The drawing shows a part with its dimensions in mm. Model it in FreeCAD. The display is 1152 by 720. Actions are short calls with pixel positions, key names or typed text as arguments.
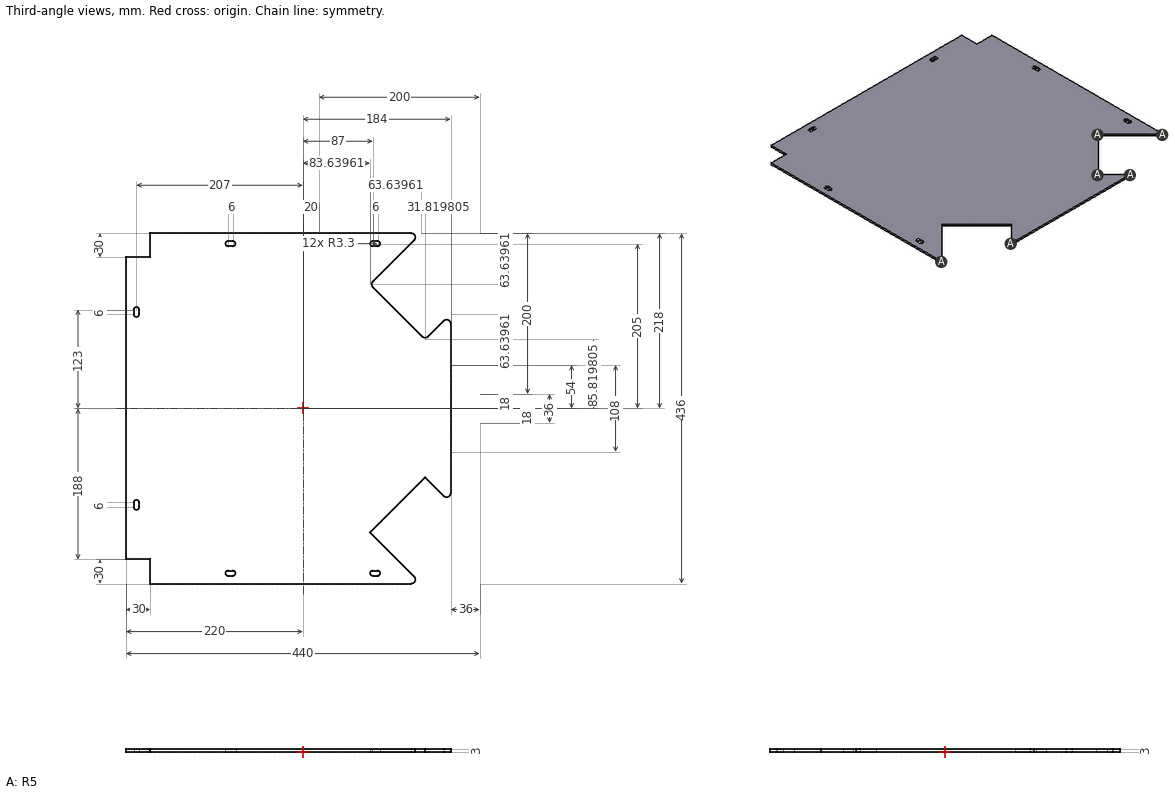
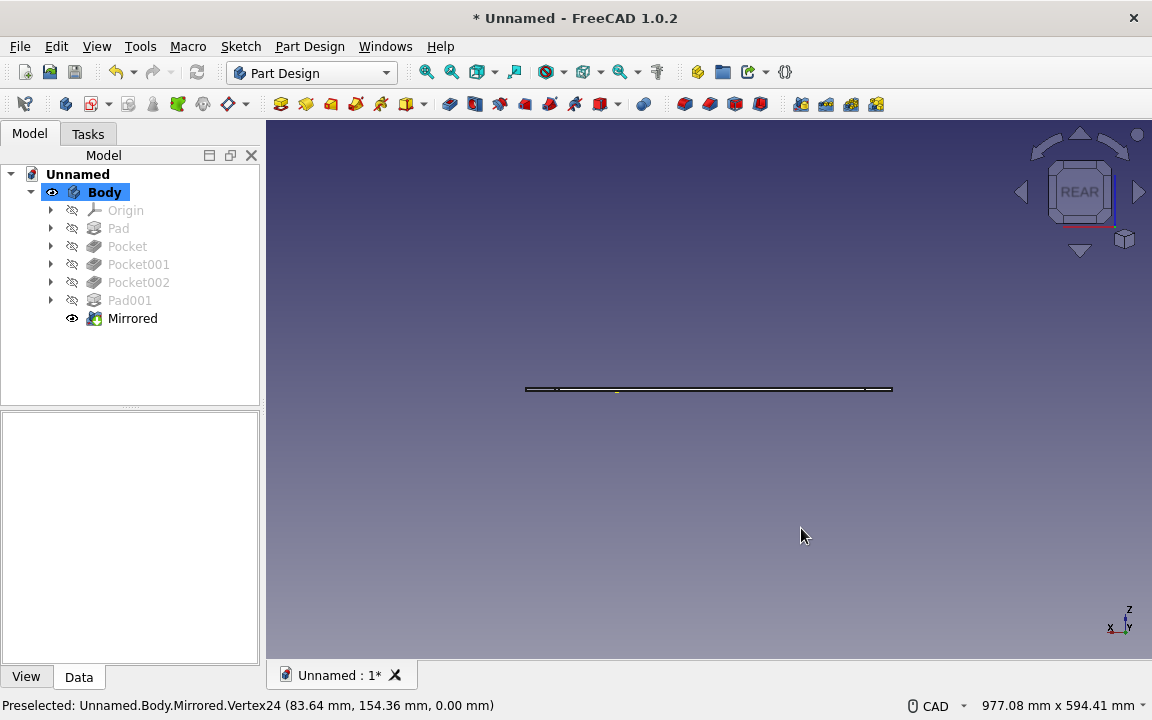
scroll(617, 389, up, 14)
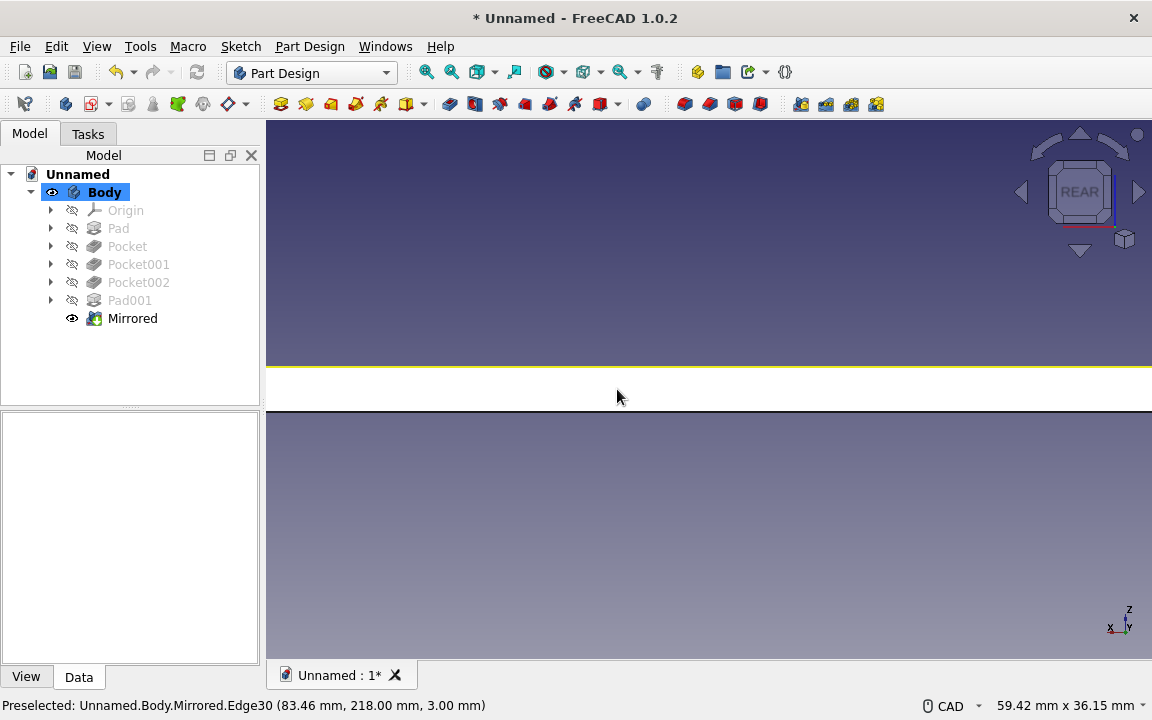
key(v)
key(f)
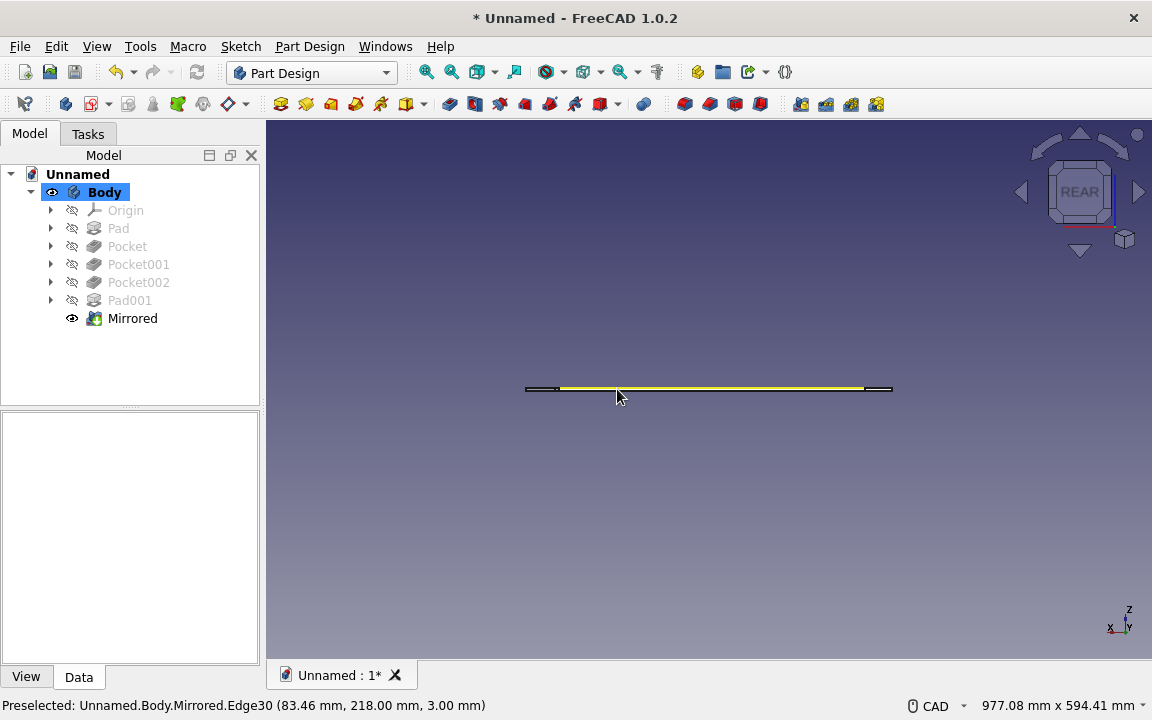
key(6)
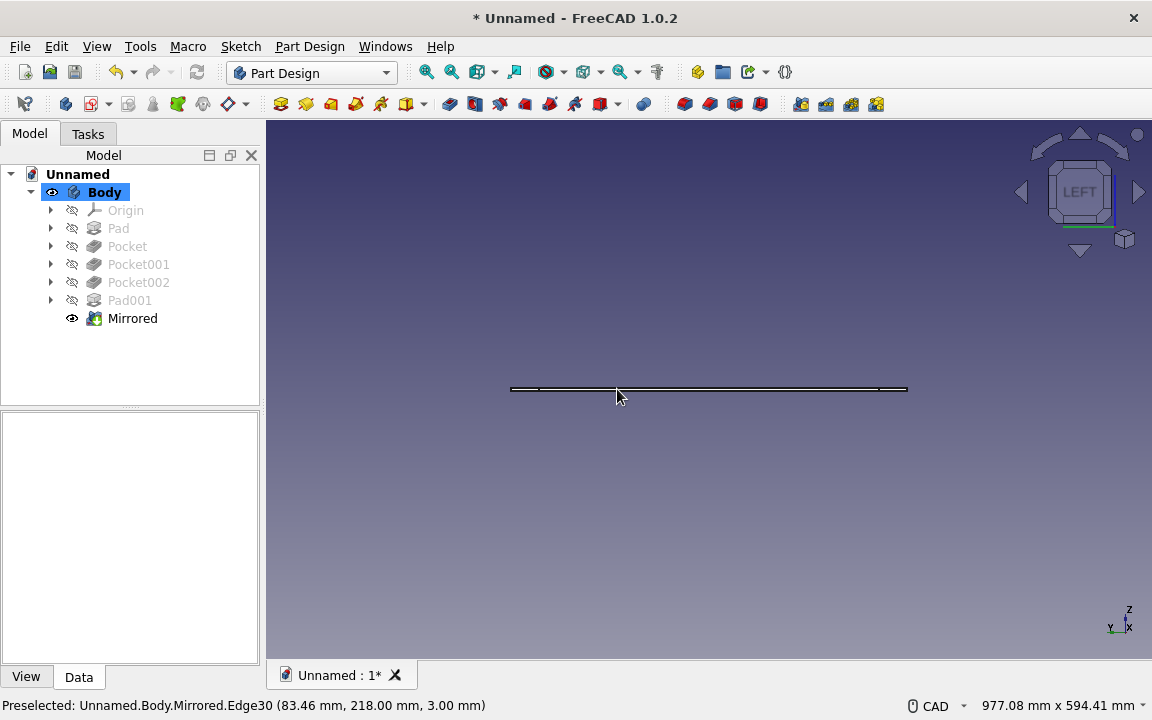
key(v)
key(f)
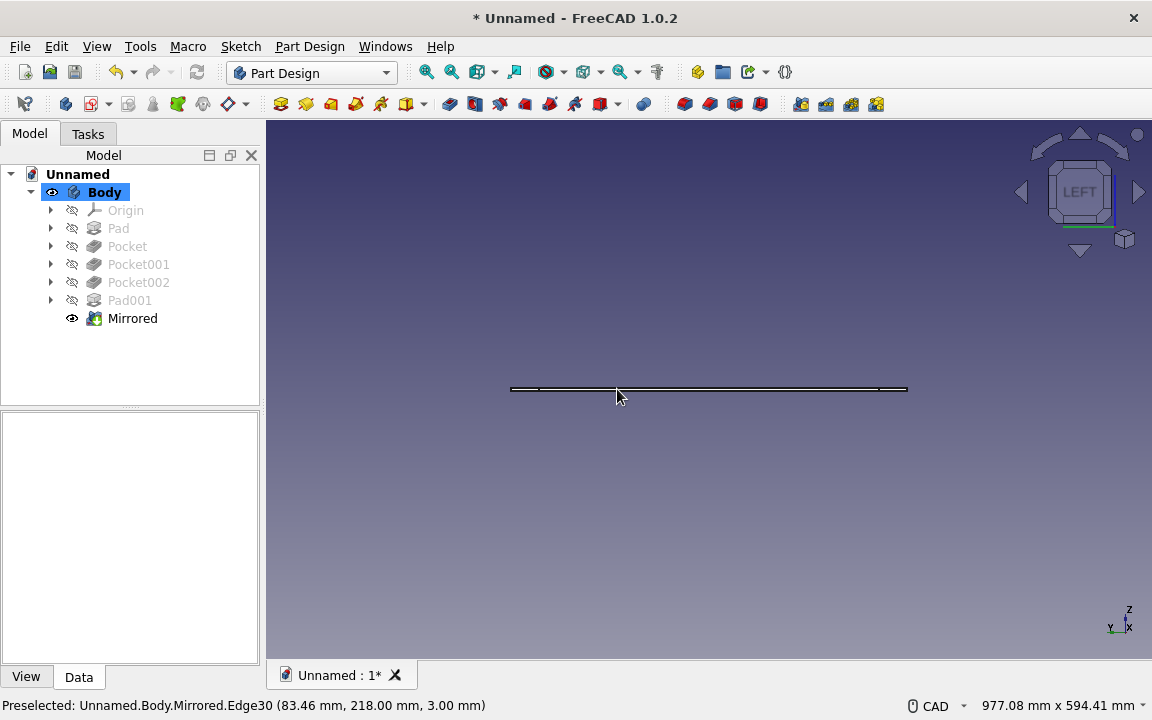
scroll(569, 388, up, 14)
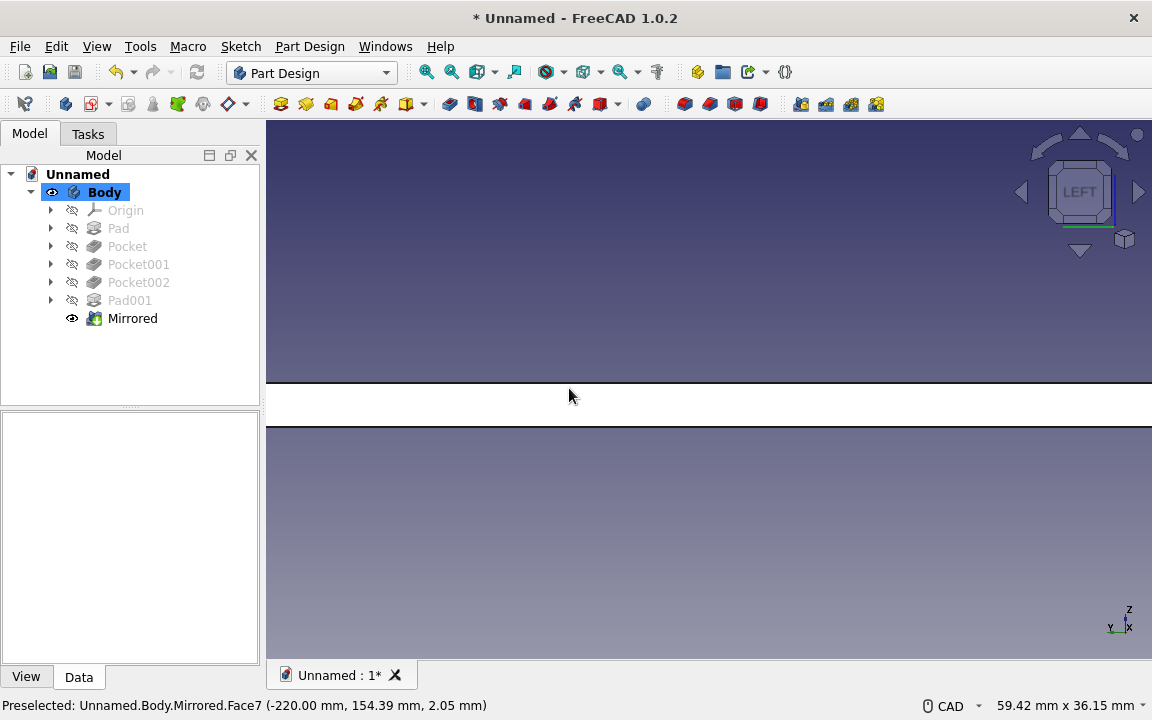
key(v)
key(f)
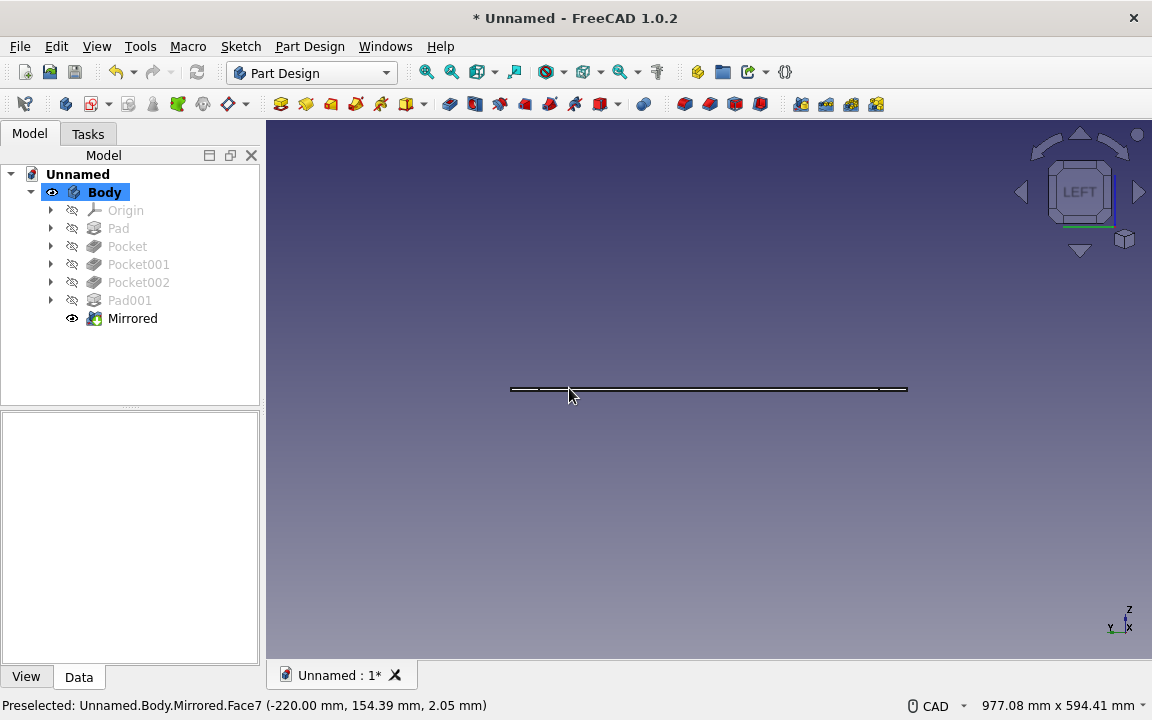
key(v)
key(3)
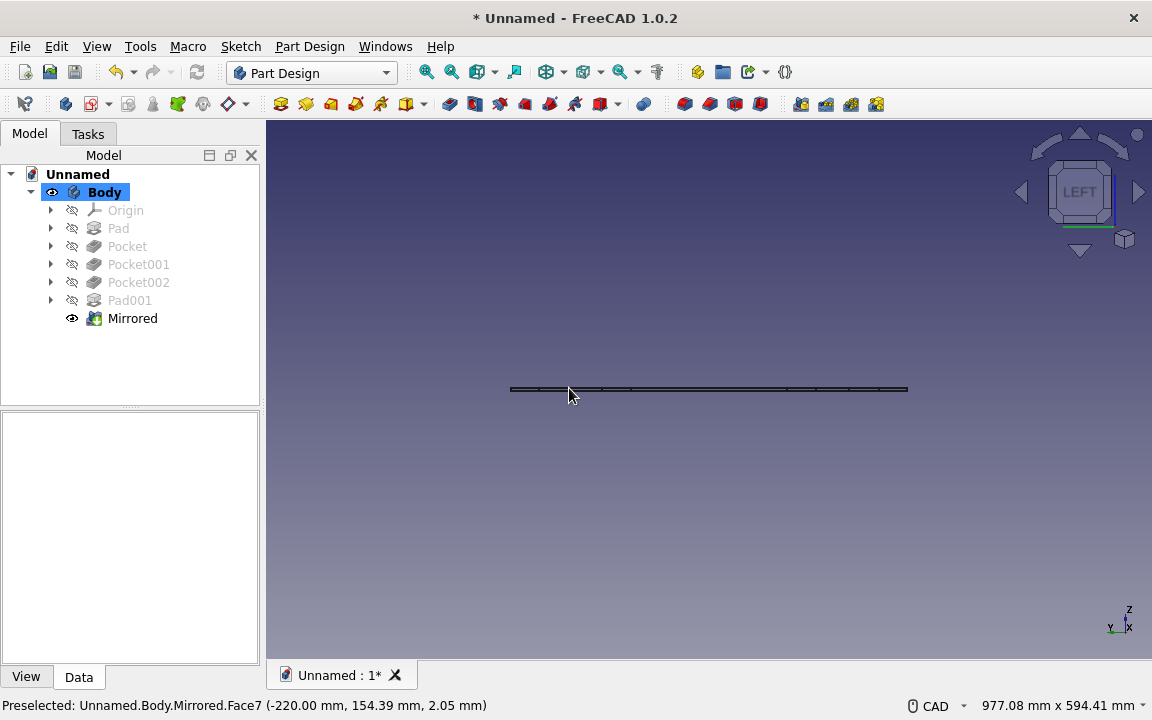
key(0)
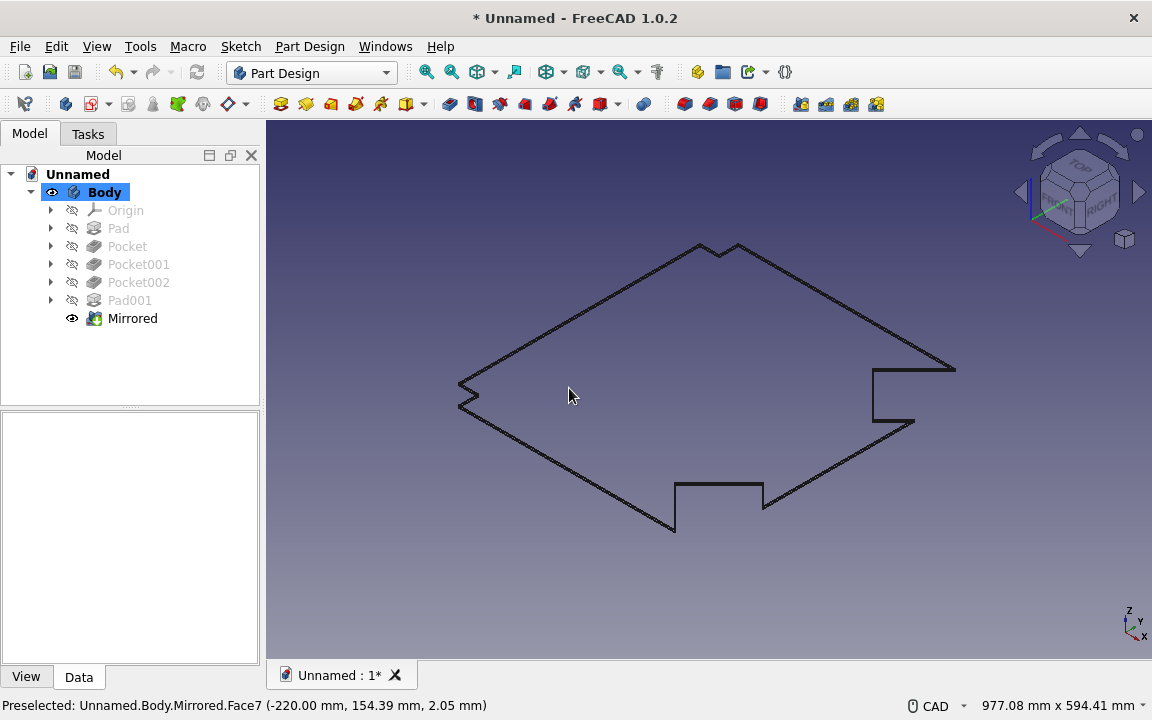
scroll(873, 369, up, 14)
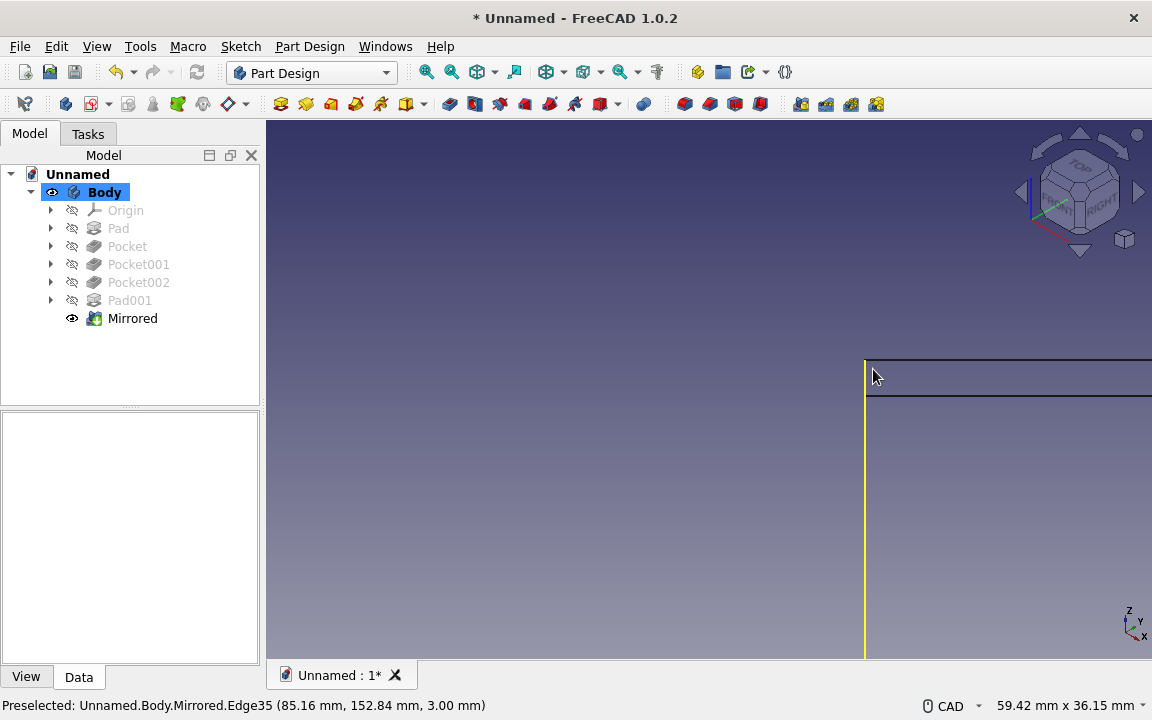
click(427, 72)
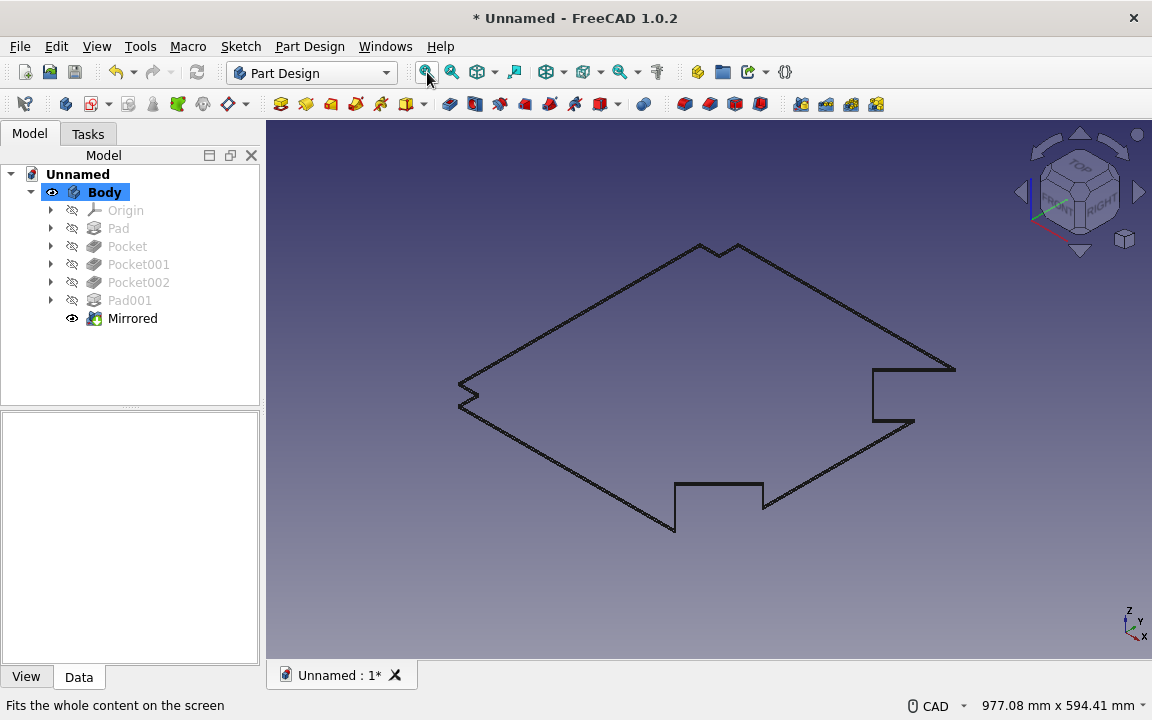
key(2)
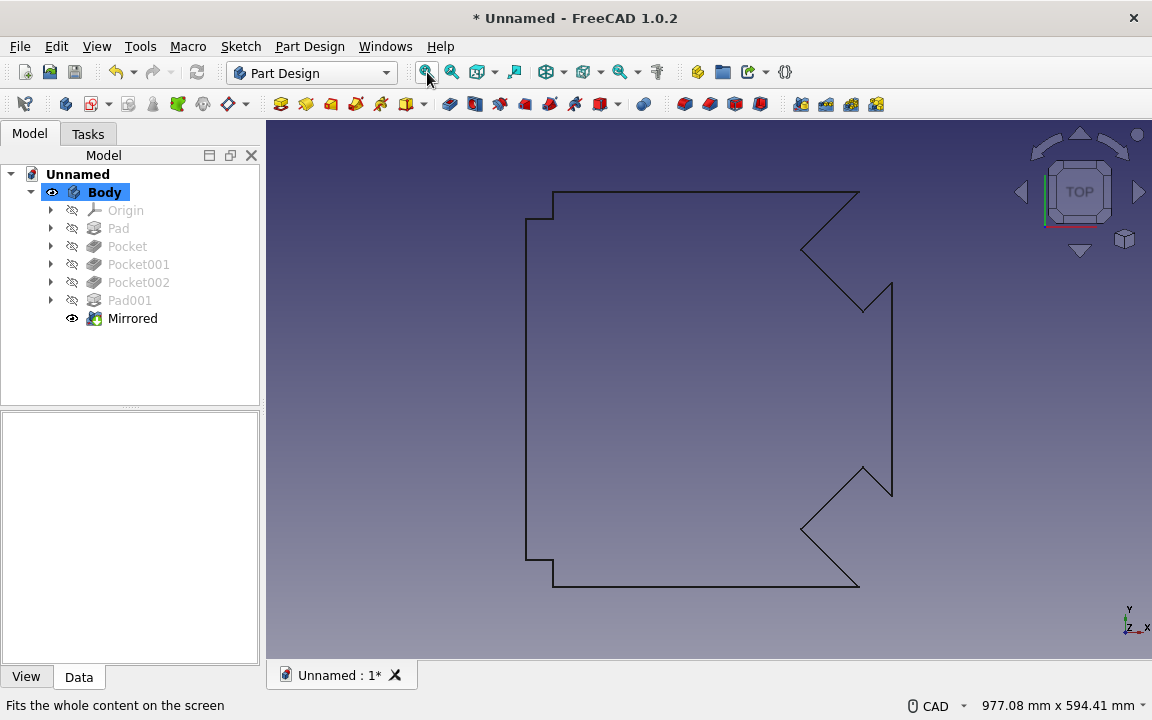
scroll(801, 249, up, 14)